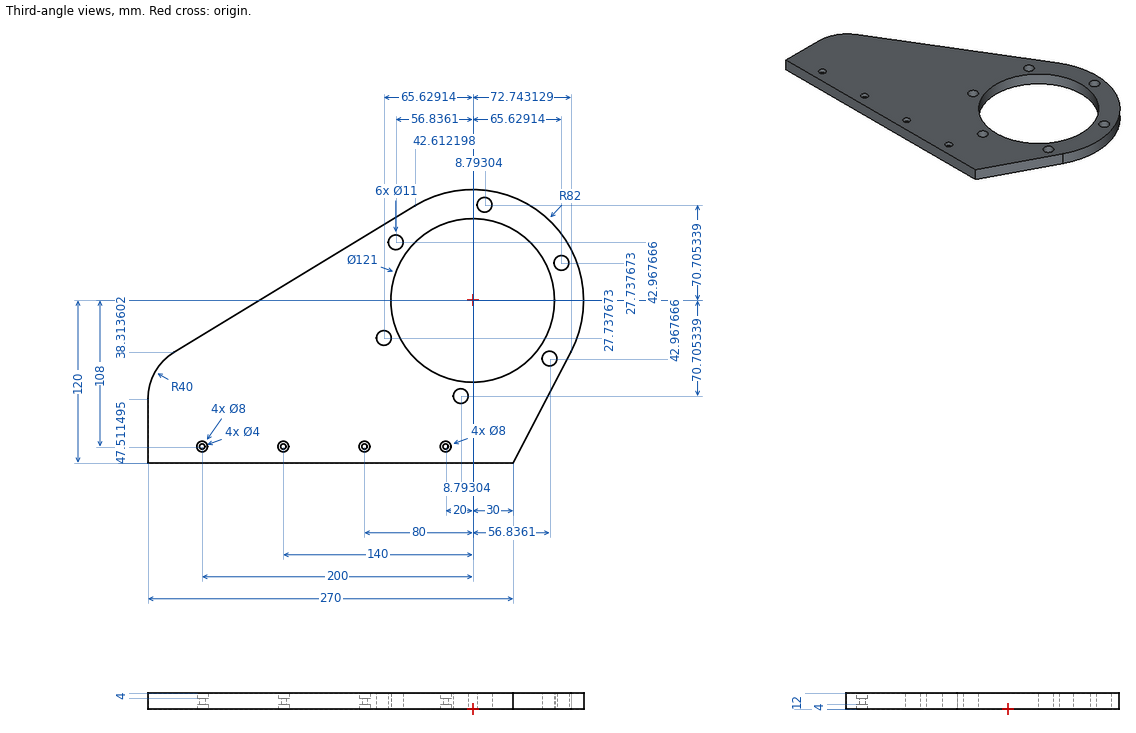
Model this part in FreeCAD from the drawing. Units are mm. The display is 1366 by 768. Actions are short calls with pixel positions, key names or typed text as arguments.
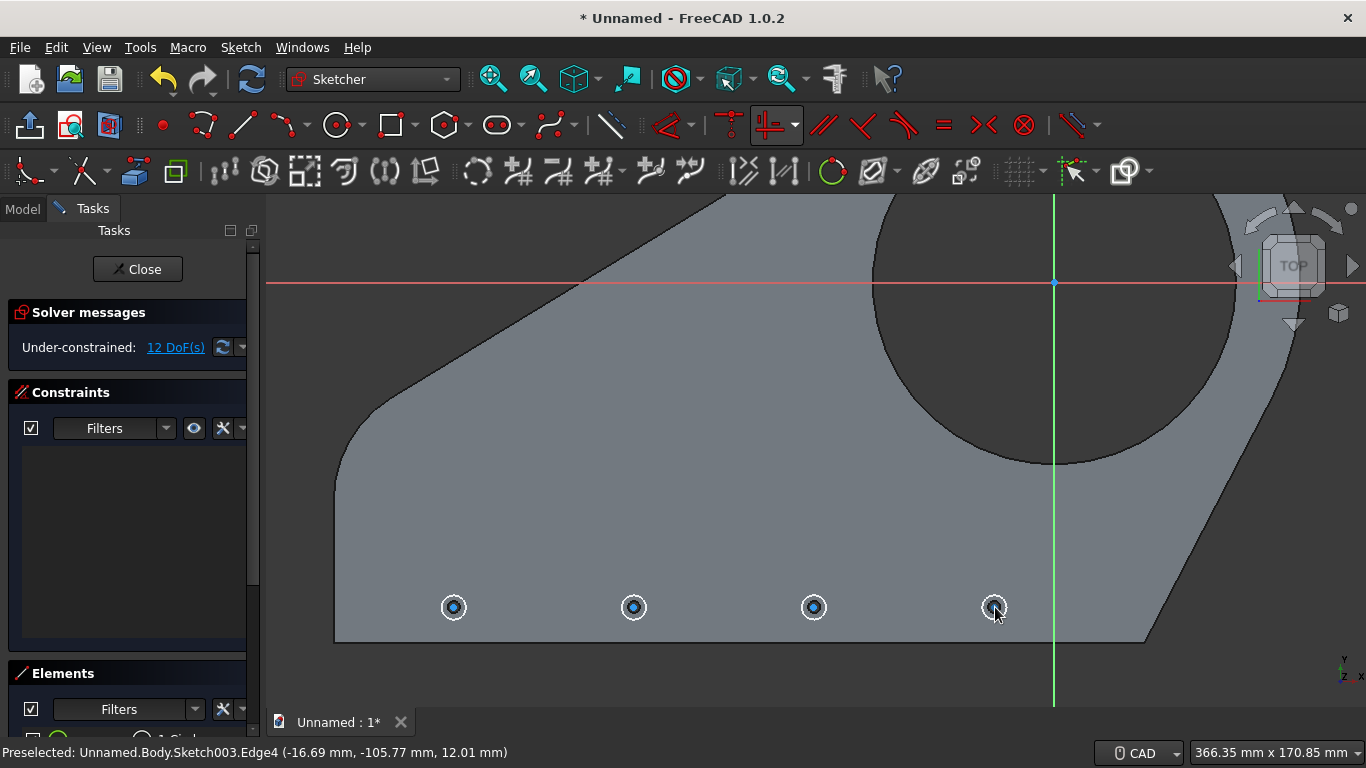
click(462, 599)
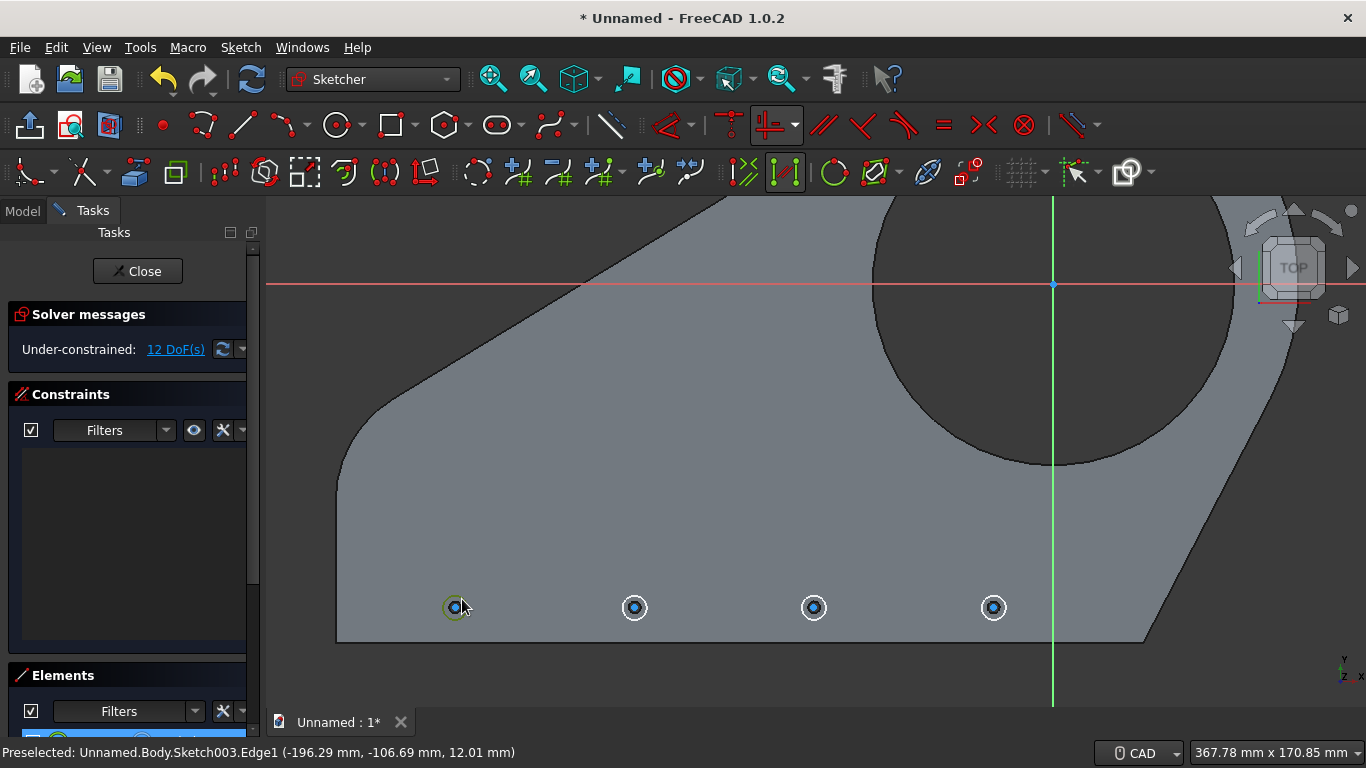
click(643, 599)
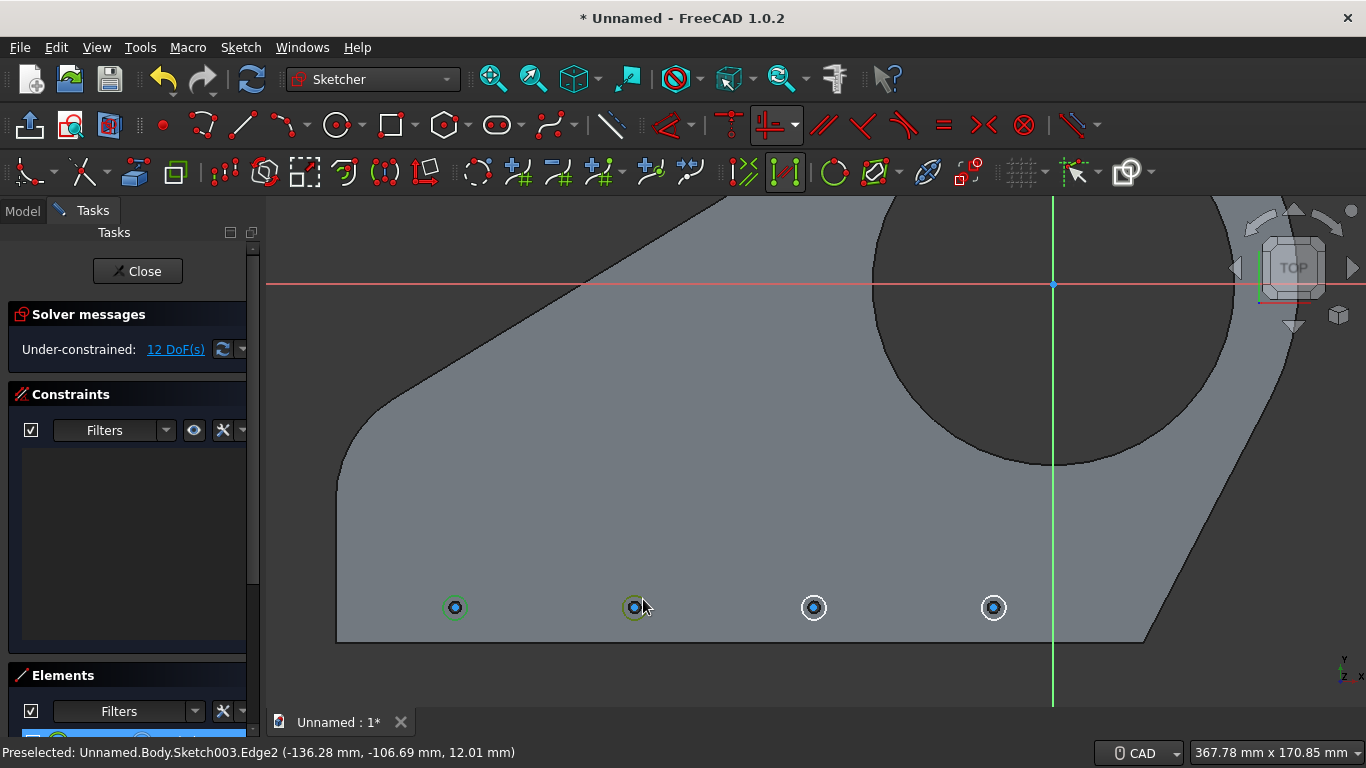
click(822, 599)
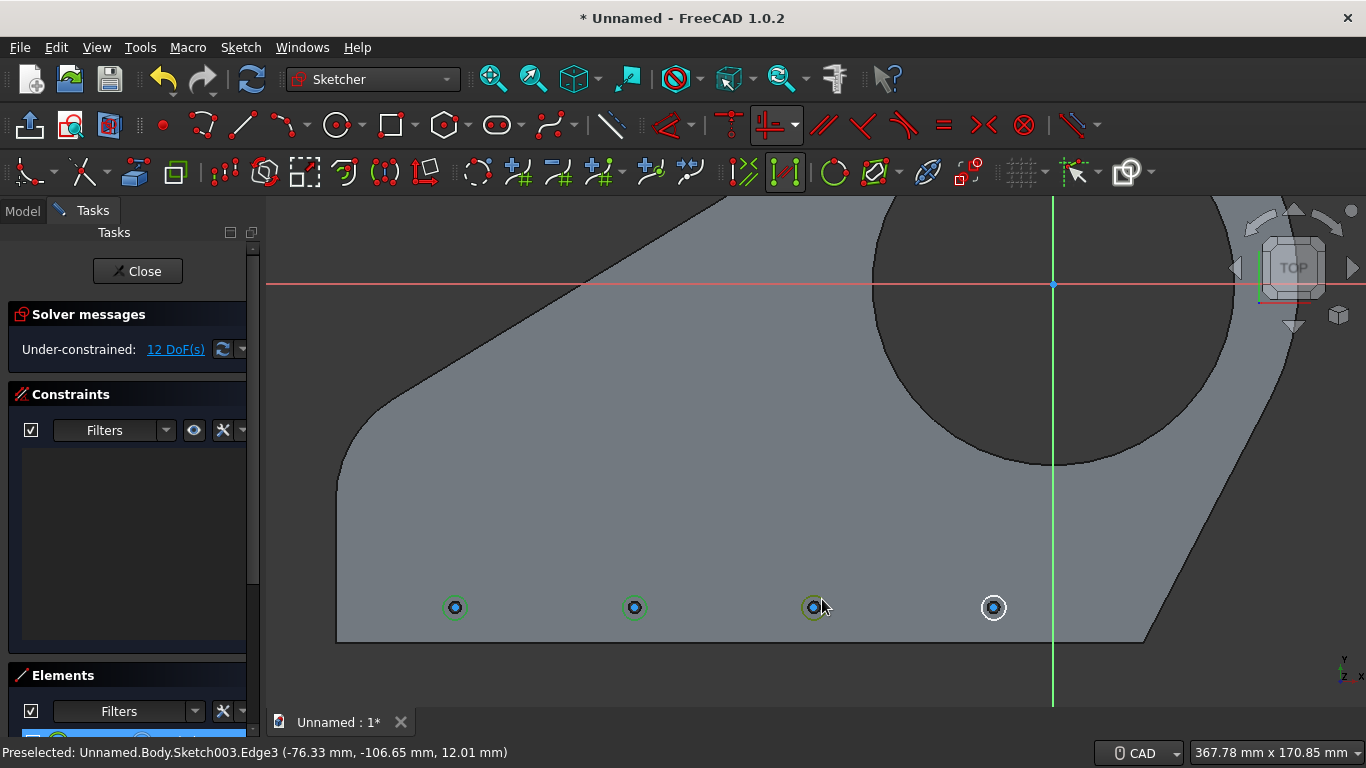
click(1002, 599)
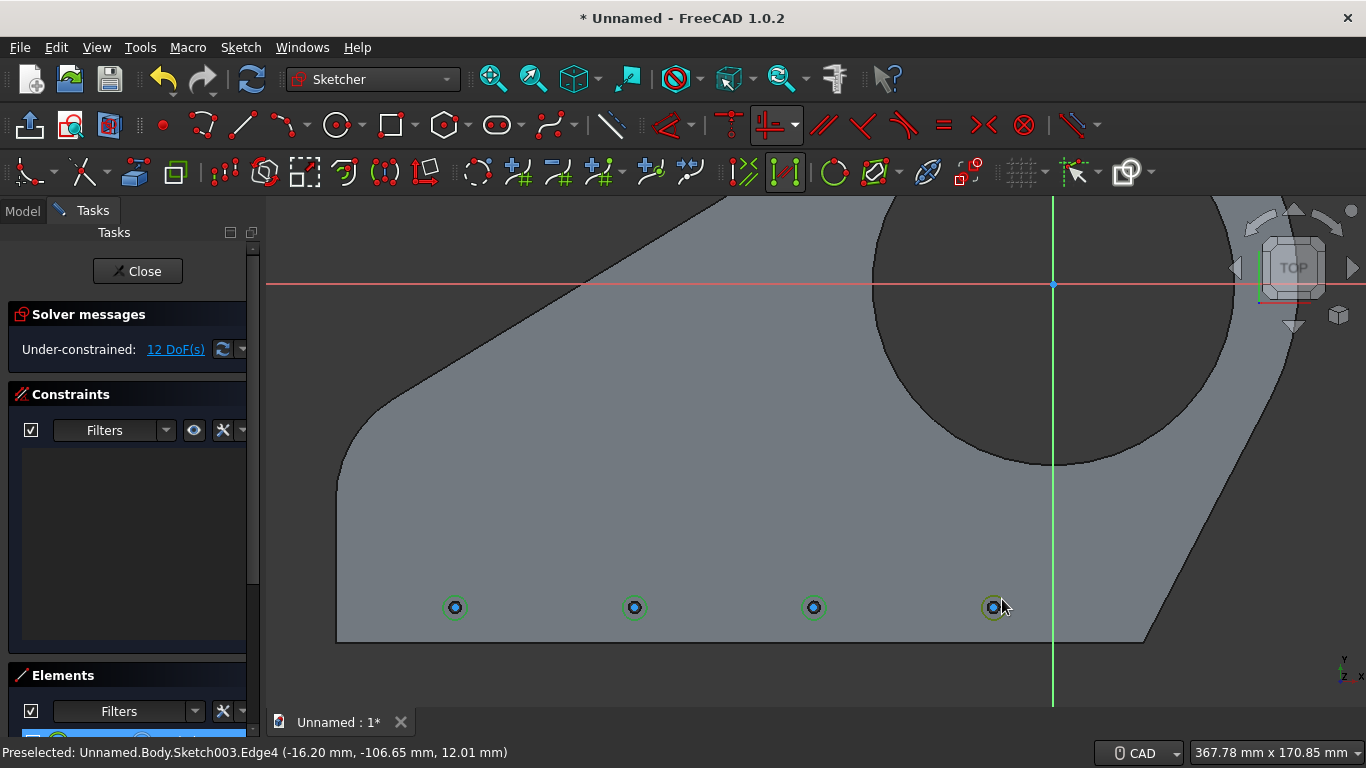
click(944, 126)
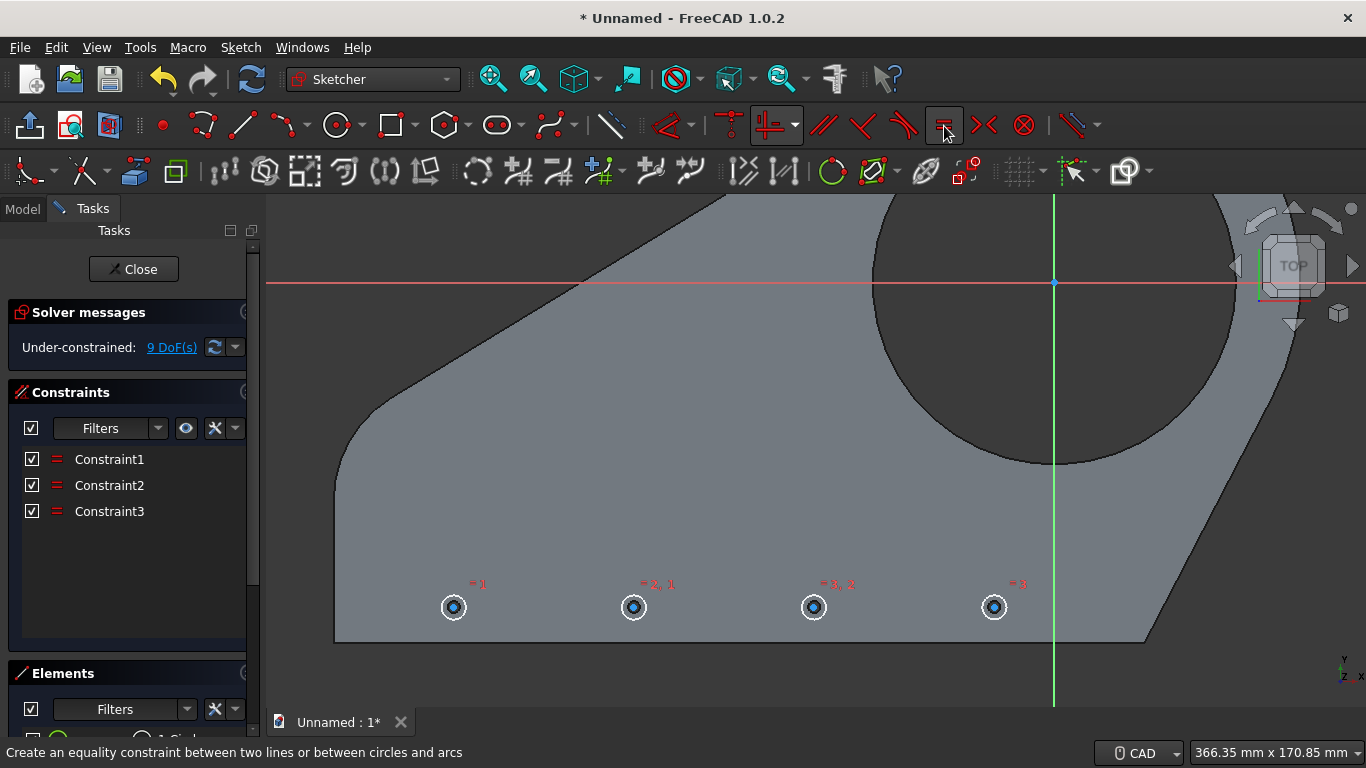
click(454, 608)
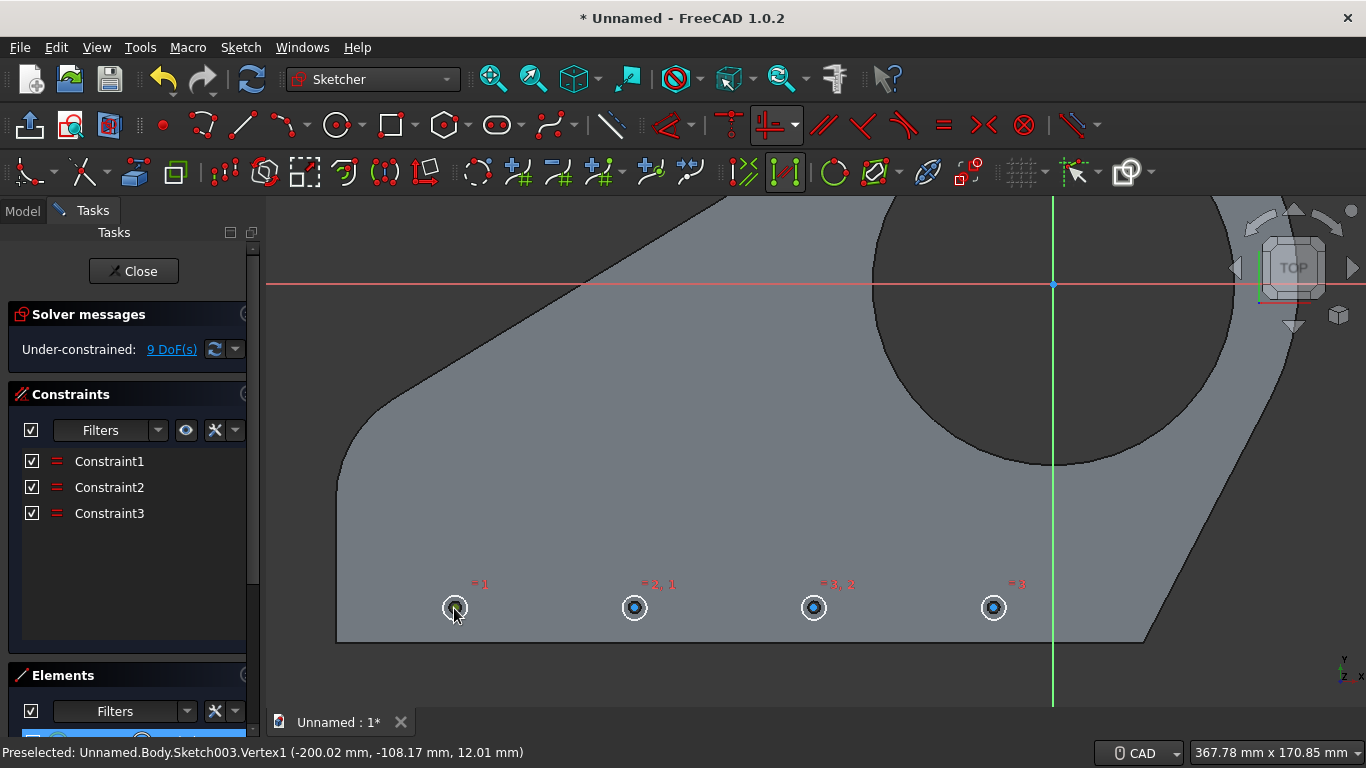
click(635, 608)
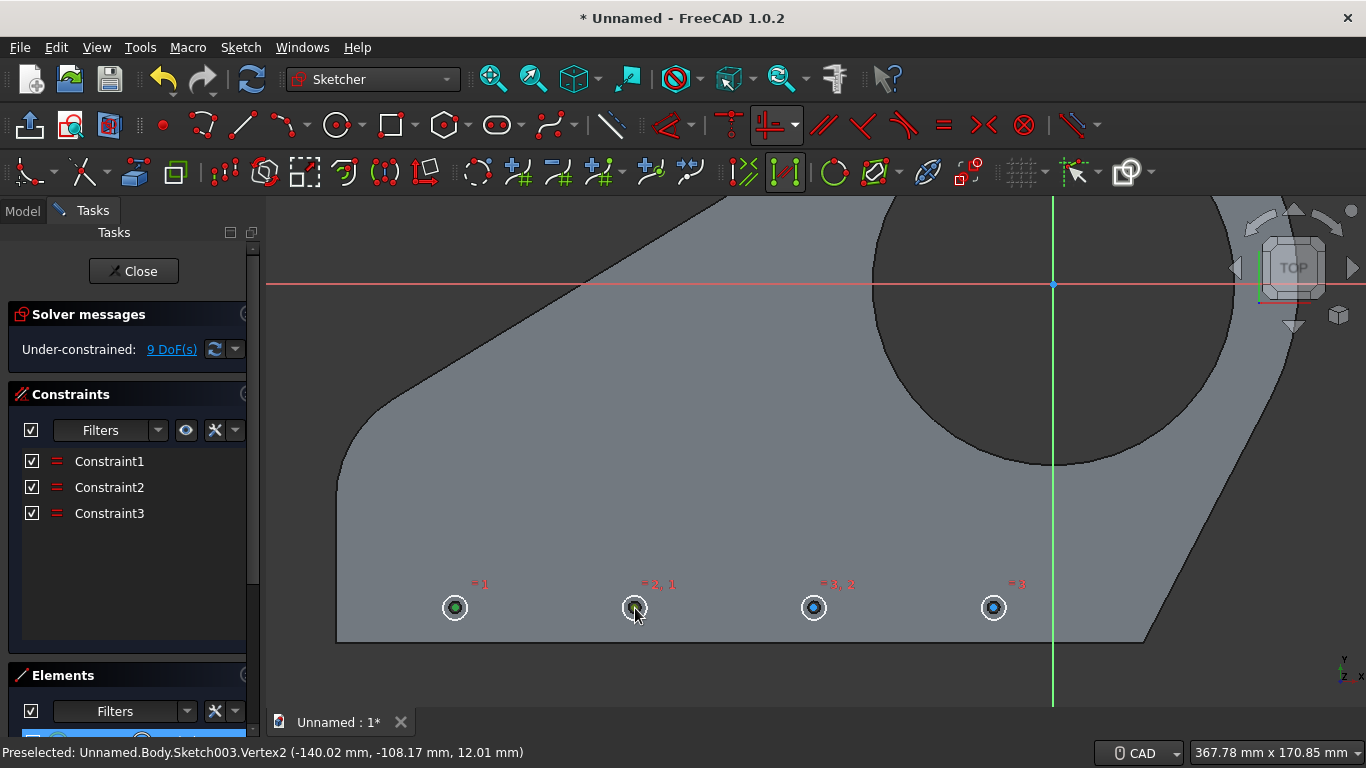
key(h)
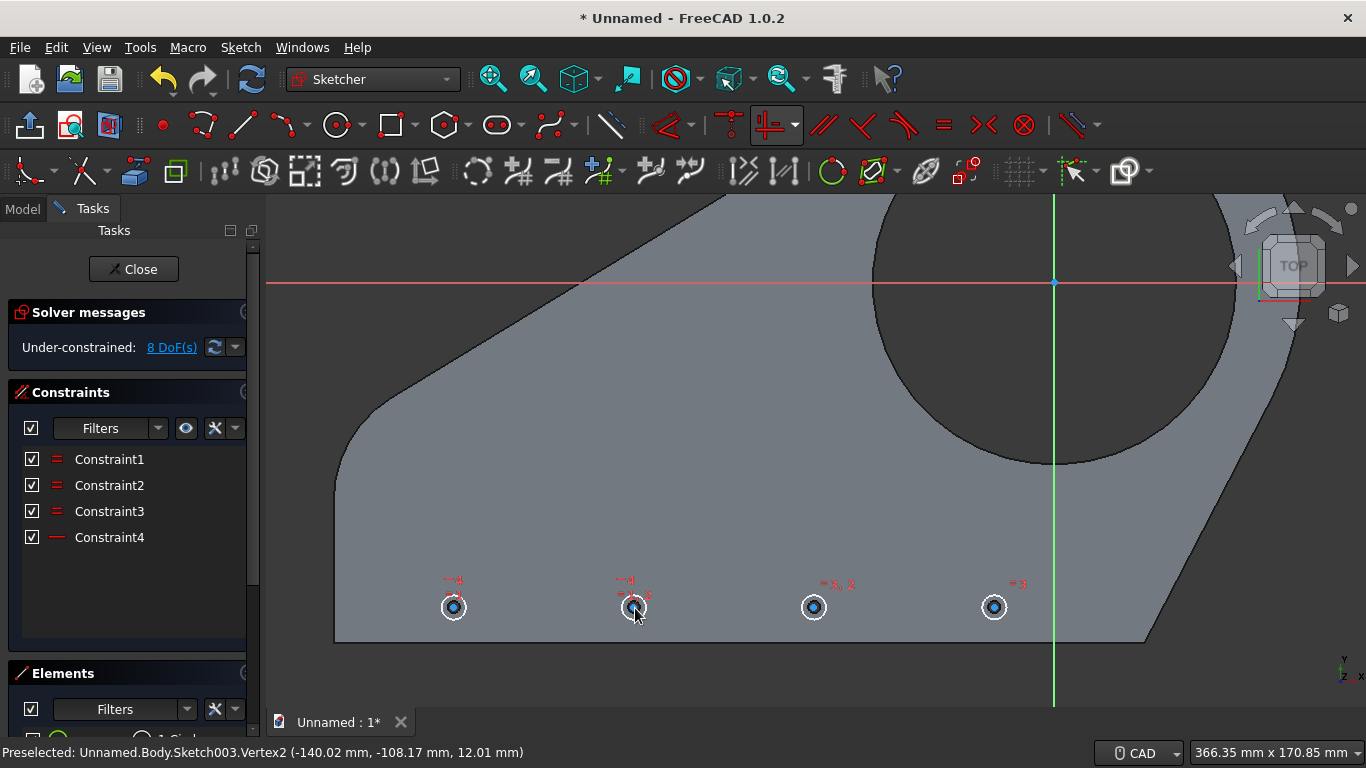
click(634, 608)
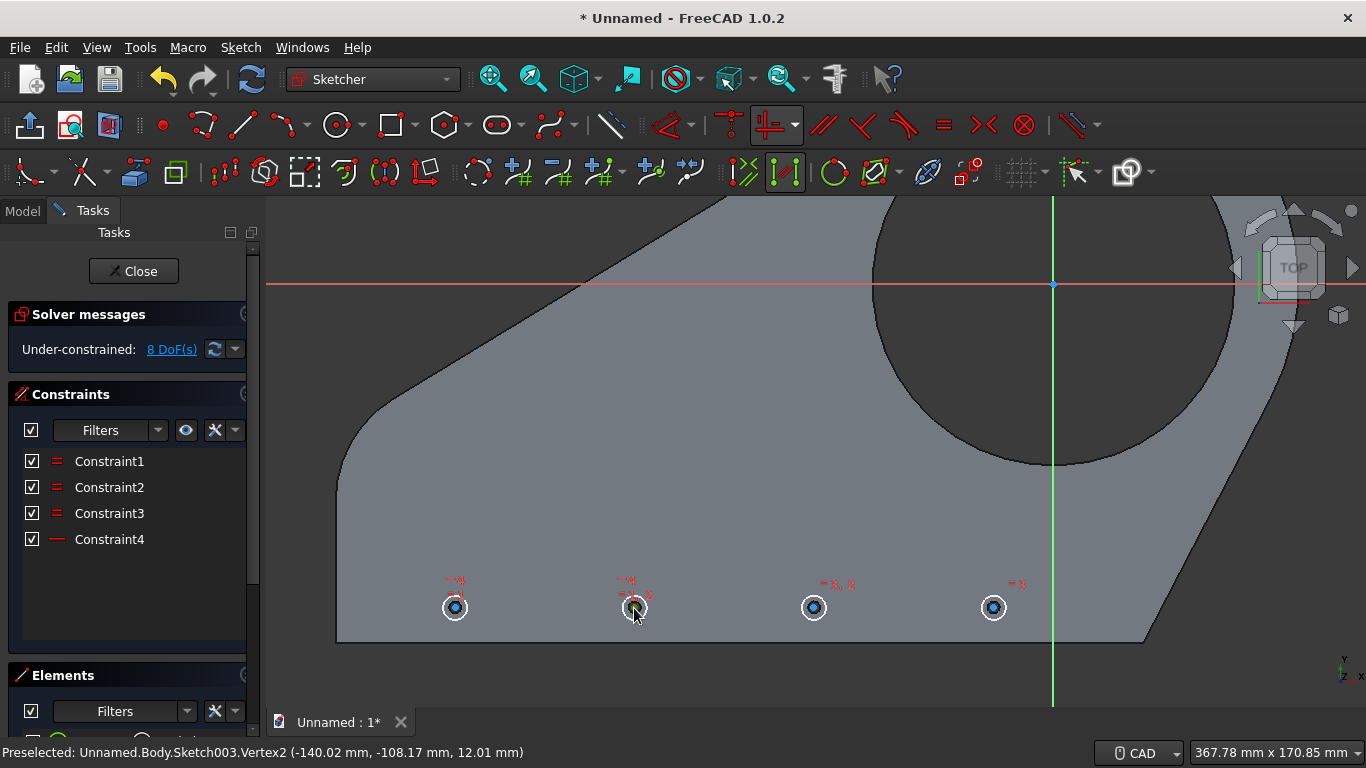
click(814, 608)